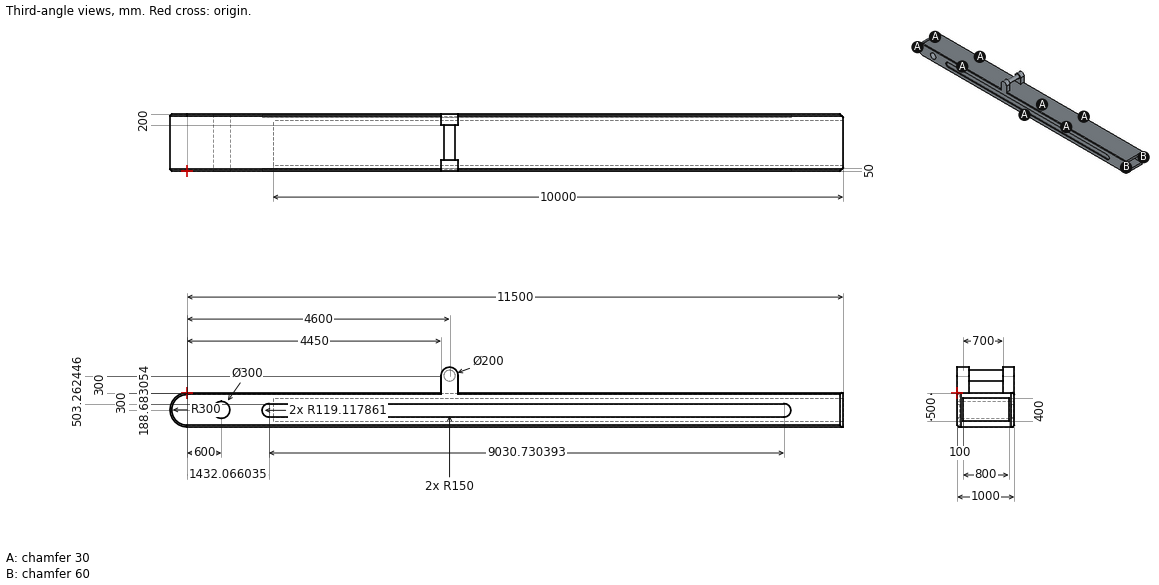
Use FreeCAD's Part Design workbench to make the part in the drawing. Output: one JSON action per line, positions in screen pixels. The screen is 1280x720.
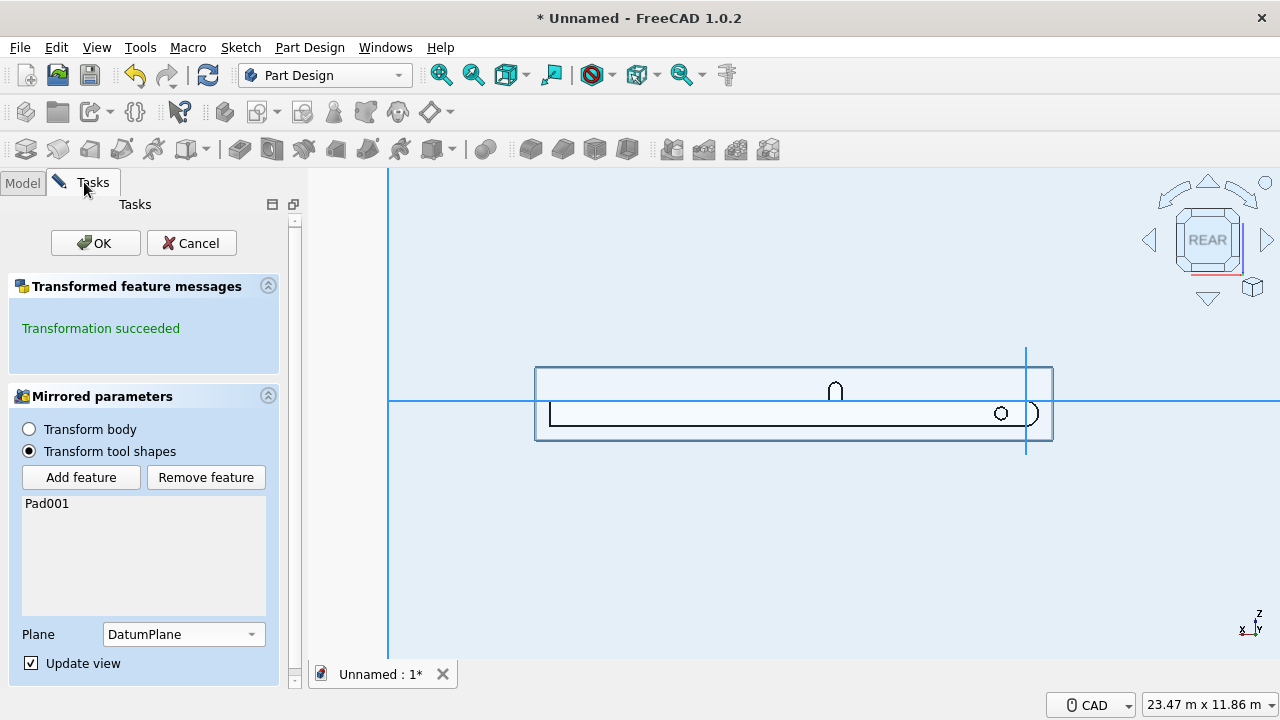
{"action": "left_click", "coordinate": [96, 243]}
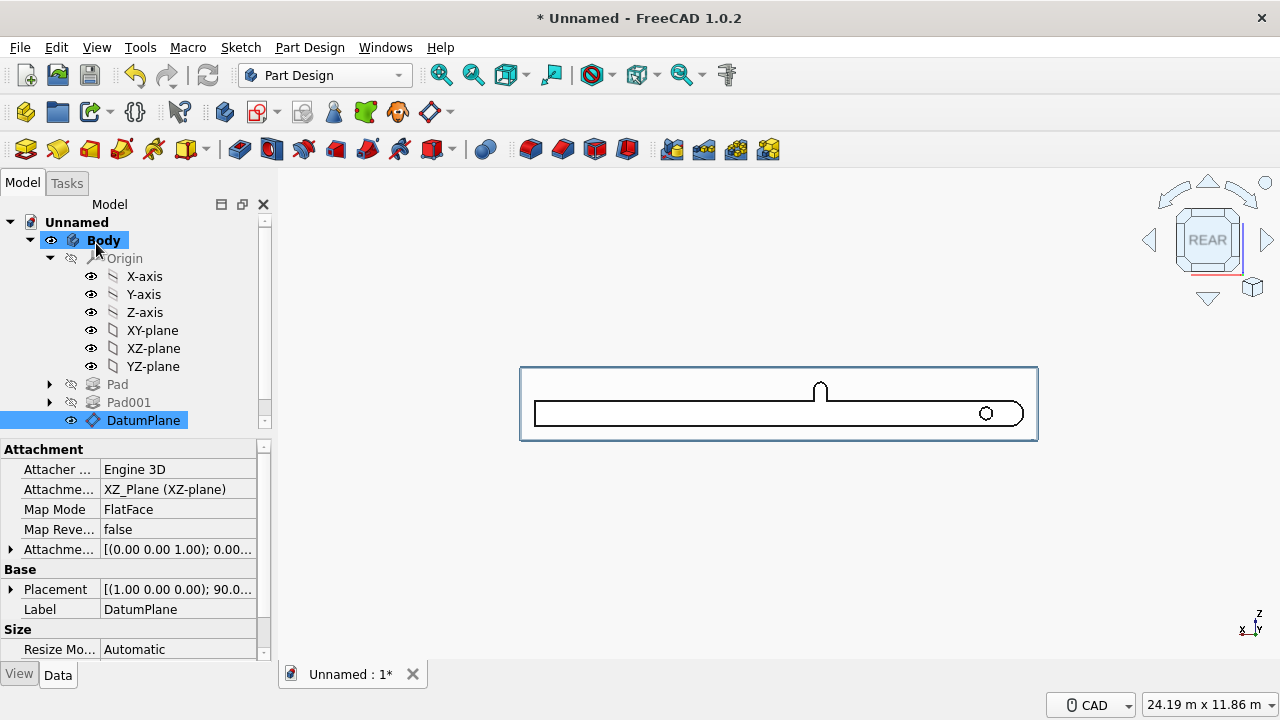
{"action": "left_click", "coordinate": [116, 420]}
{"action": "key", "text": "space"}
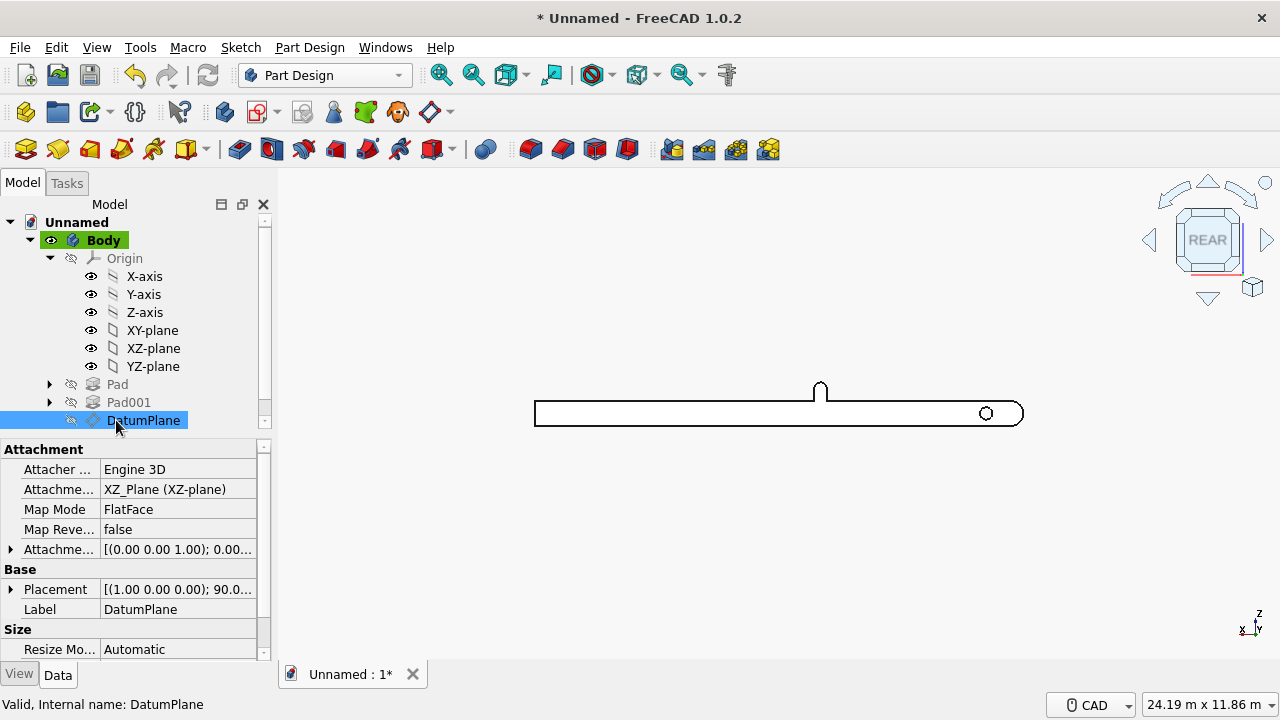
{"action": "left_click", "coordinate": [136, 348]}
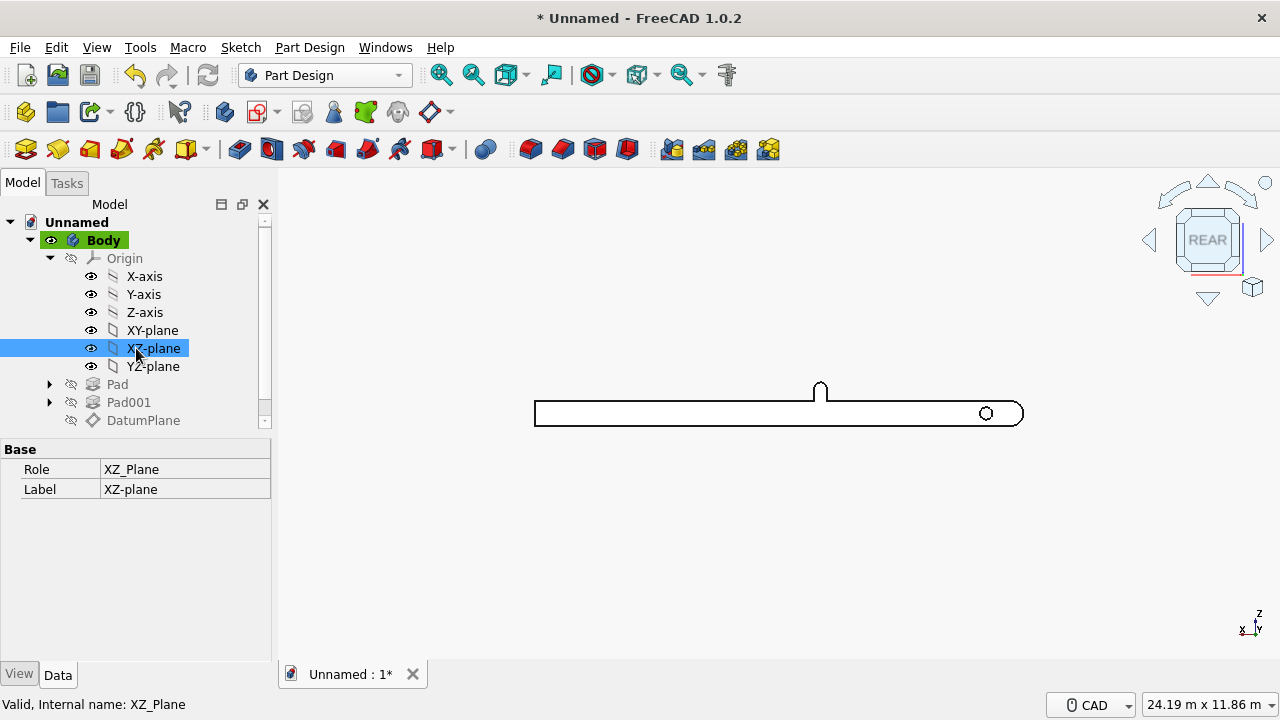
{"action": "left_click", "coordinate": [430, 112]}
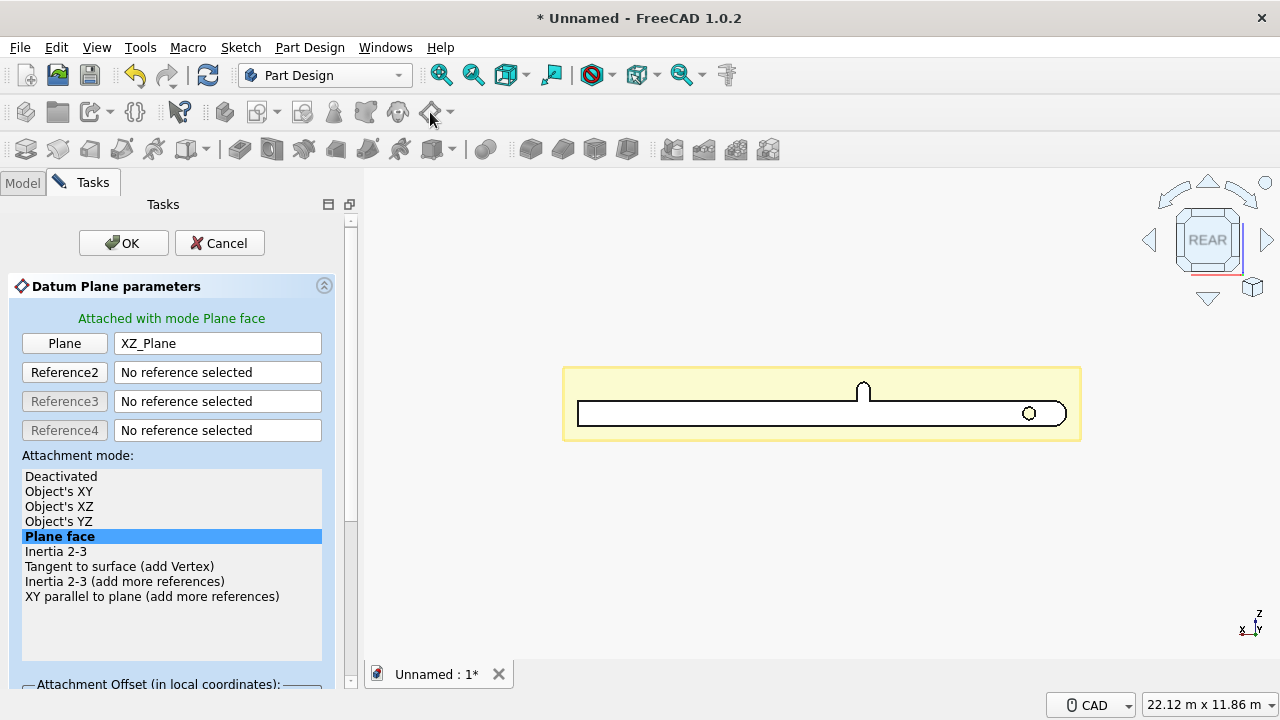
{"action": "scroll", "coordinate": [351, 451], "scroll_direction": "down", "scroll_amount": 3}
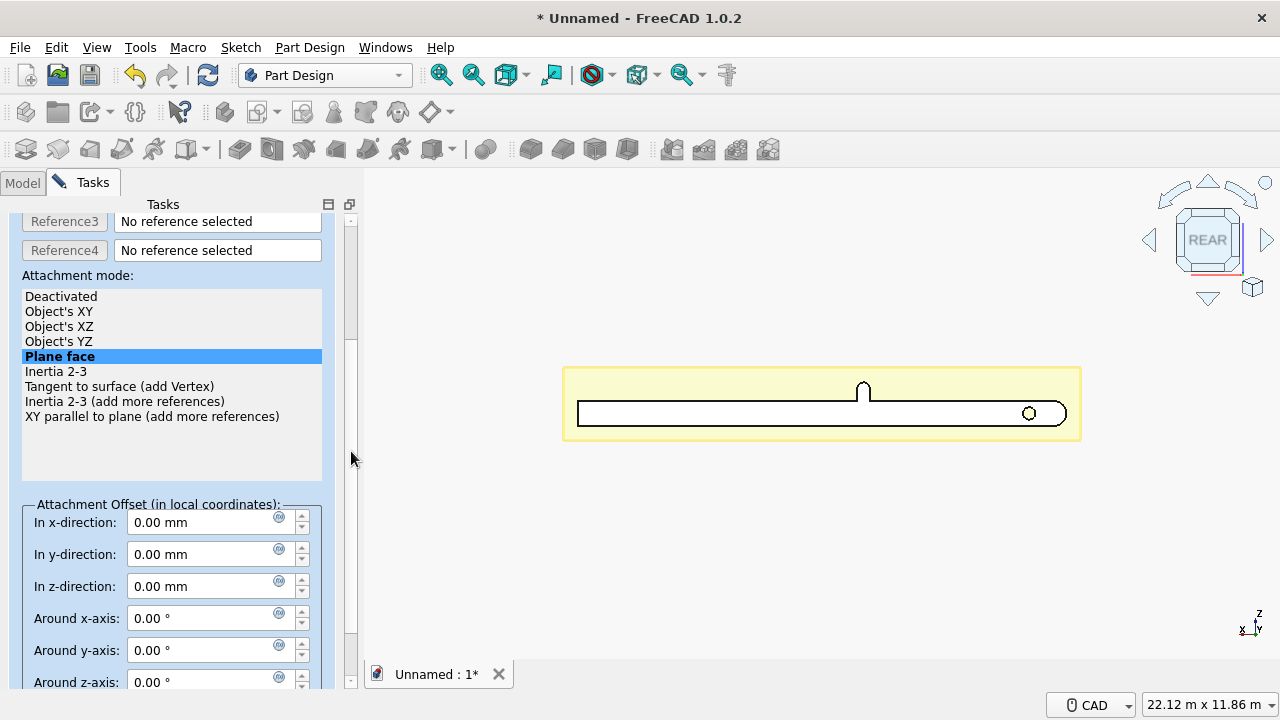
{"action": "triple_click", "coordinate": [210, 586]}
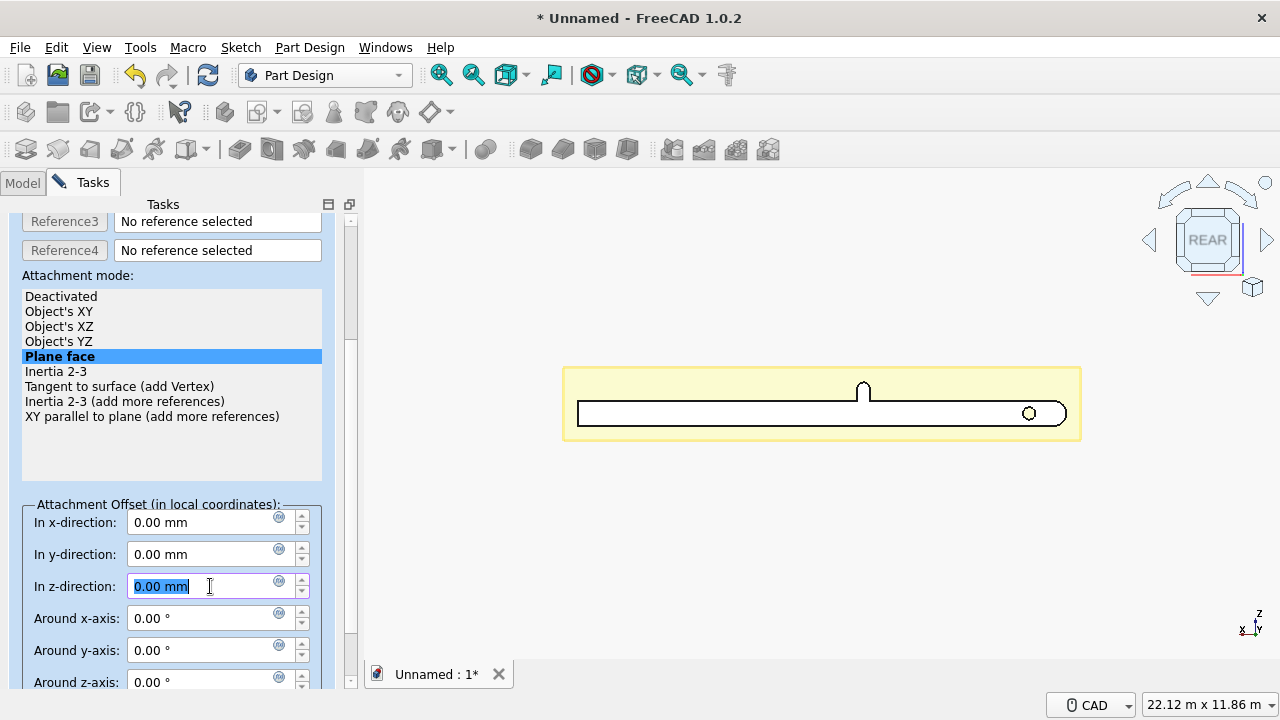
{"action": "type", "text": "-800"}
{"action": "key", "text": "Tab"}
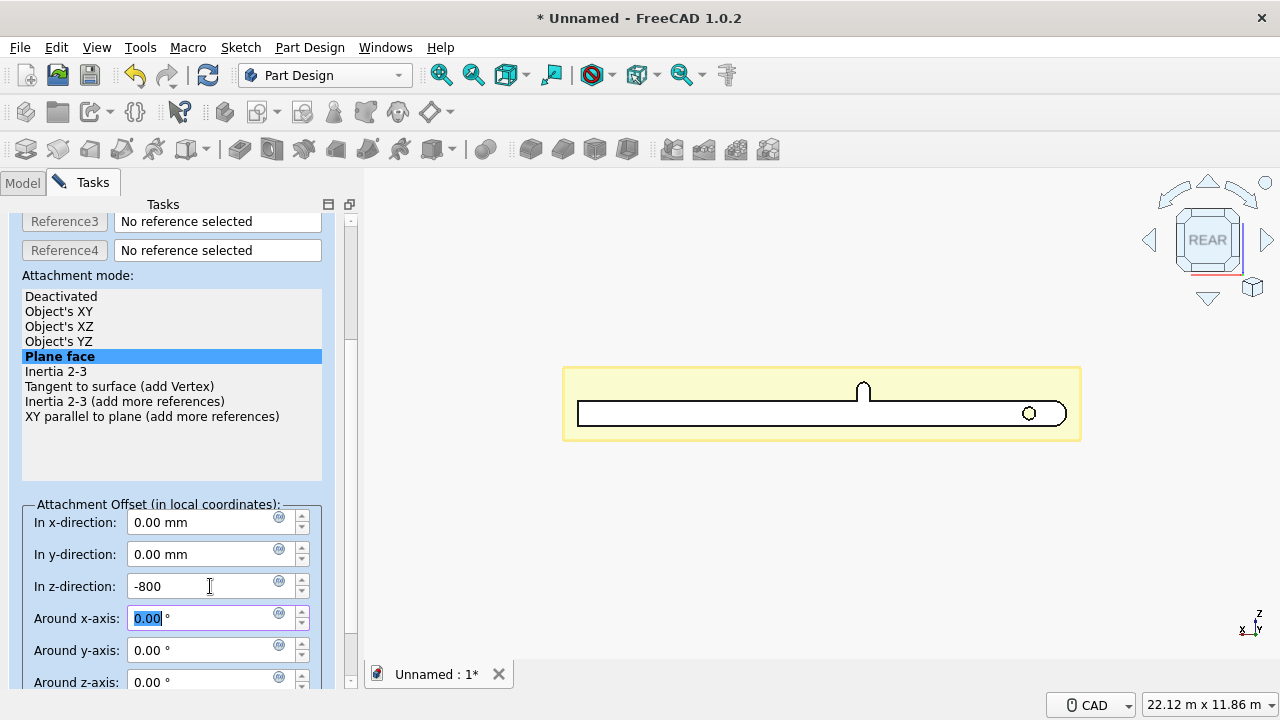
{"action": "scroll", "coordinate": [351, 451], "scroll_direction": "up", "scroll_amount": 4}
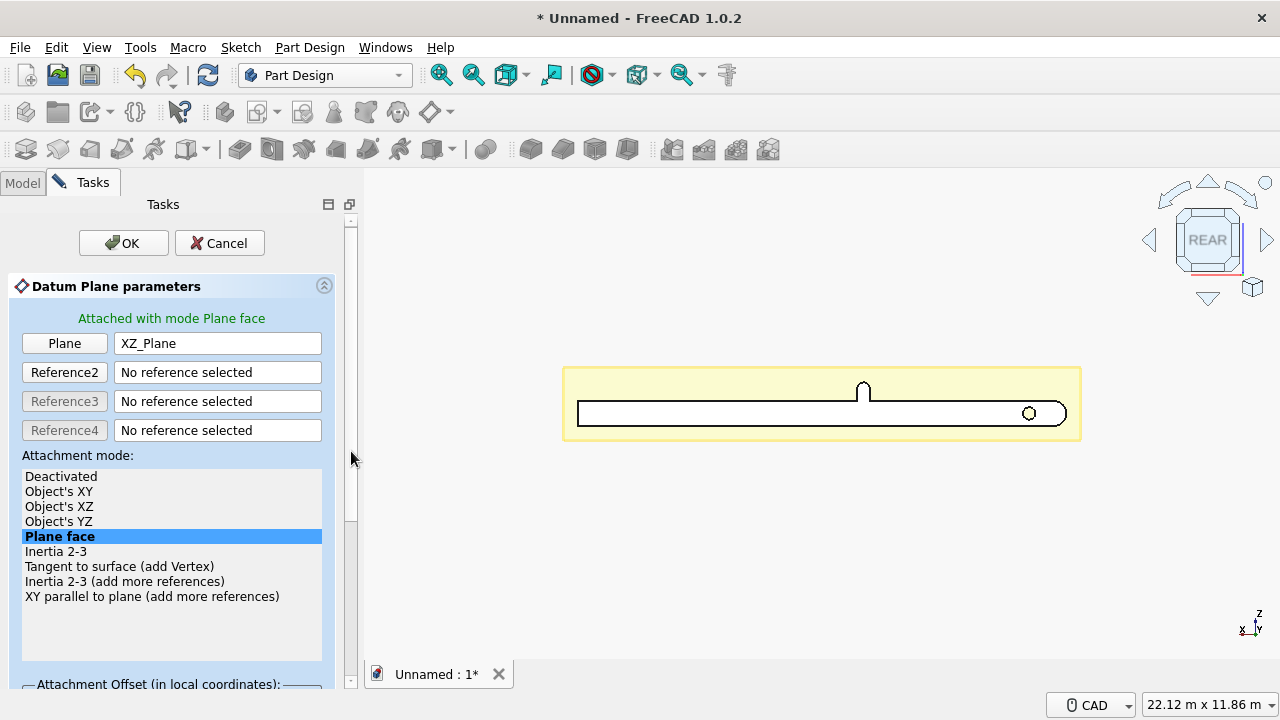
{"action": "left_click", "coordinate": [124, 243]}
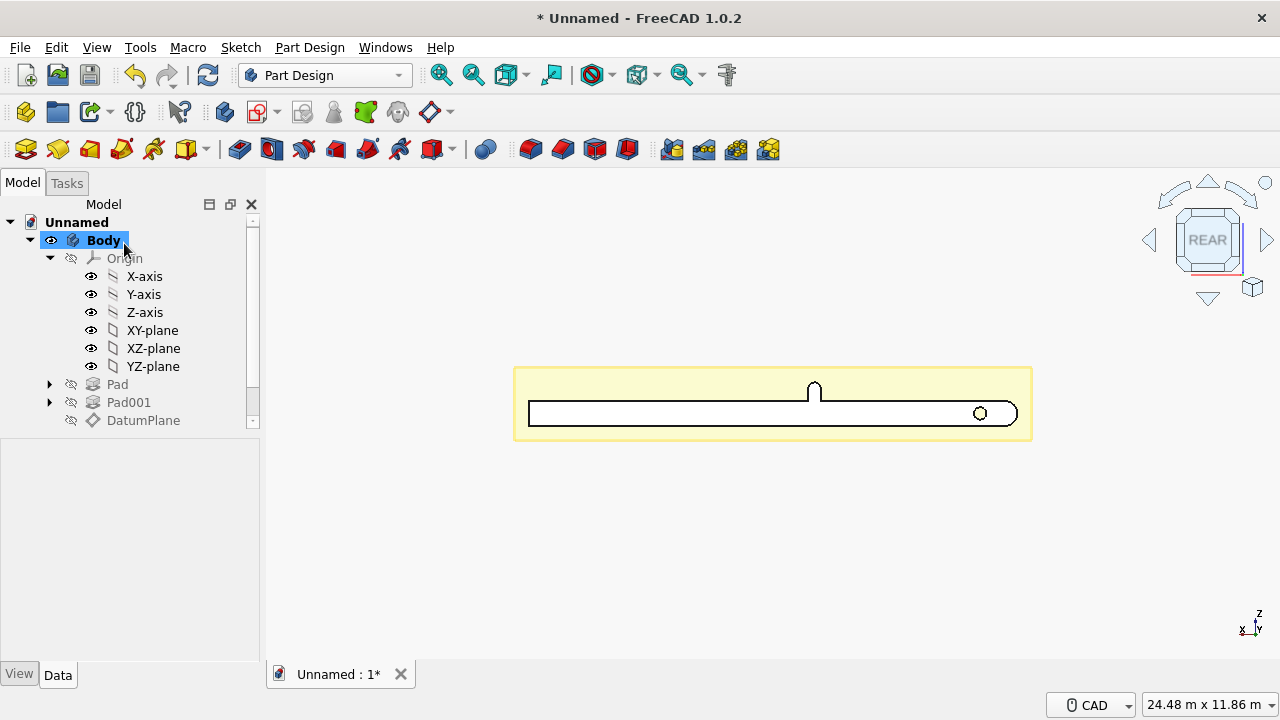
{"action": "scroll", "coordinate": [100, 326], "scroll_direction": "down", "scroll_amount": 3}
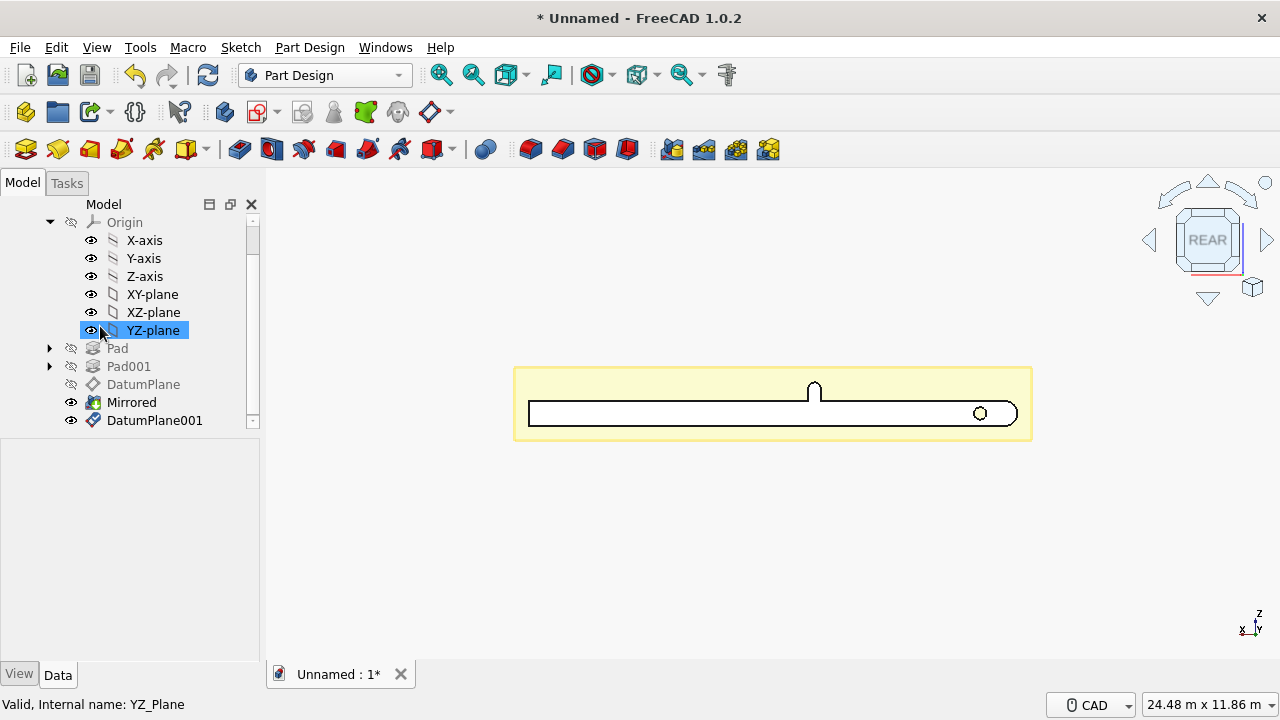
{"action": "left_click", "coordinate": [116, 420]}